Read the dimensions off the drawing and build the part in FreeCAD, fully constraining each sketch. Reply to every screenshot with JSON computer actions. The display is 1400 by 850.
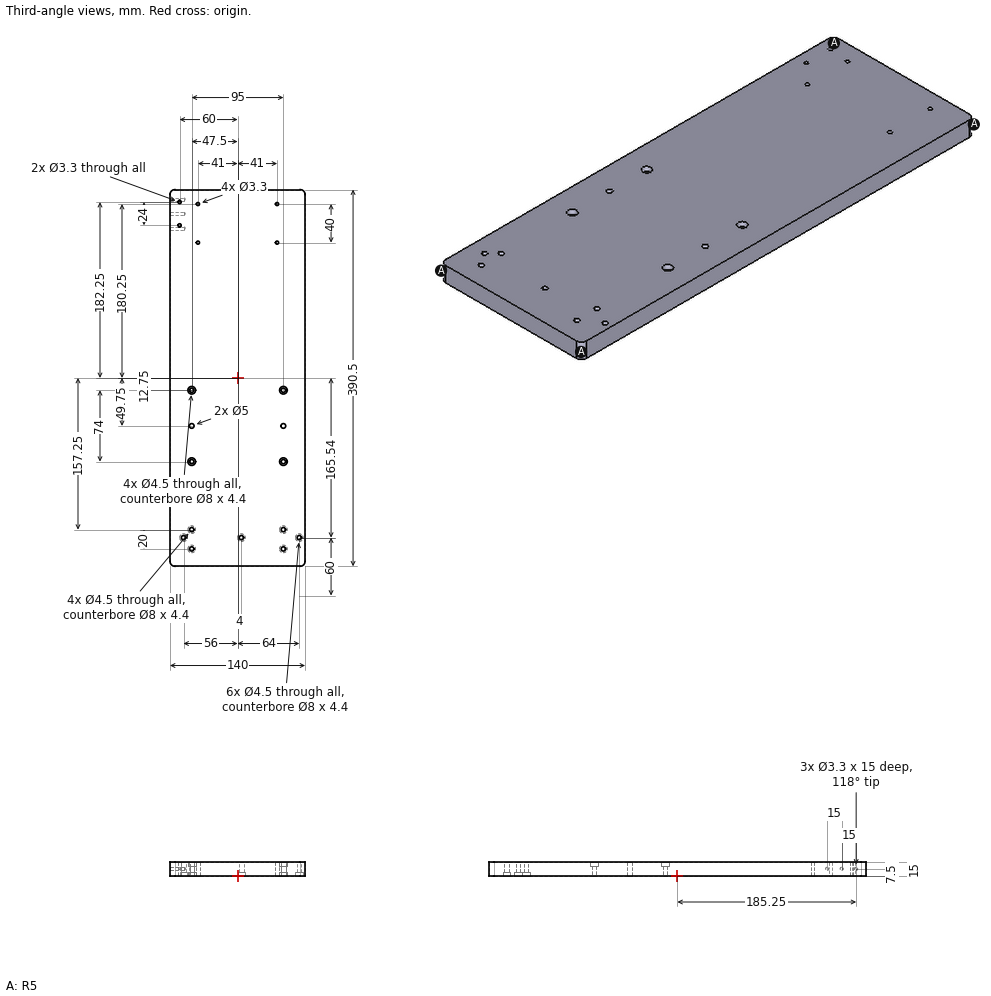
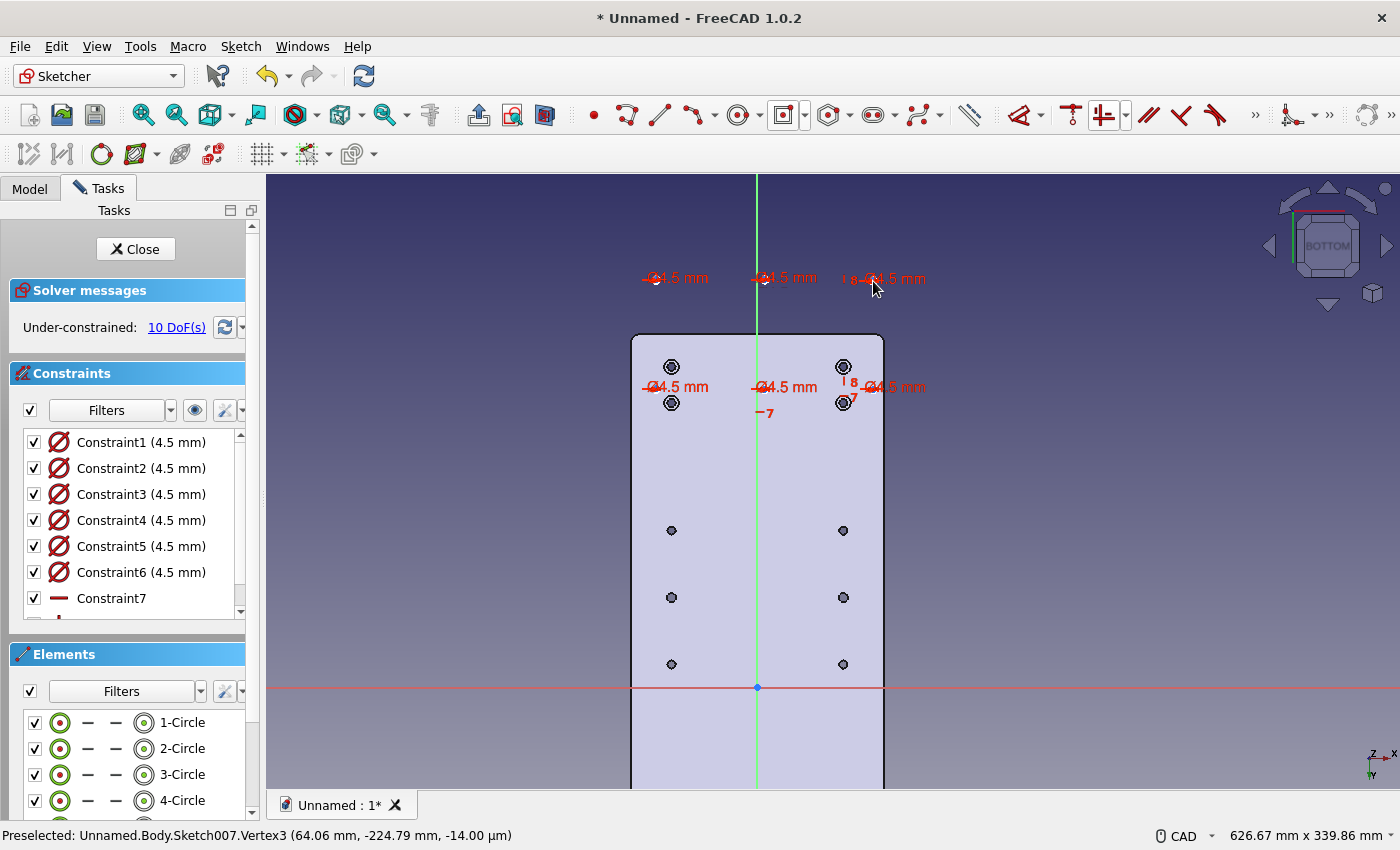
{"action": "left_click", "coordinate": [765, 389]}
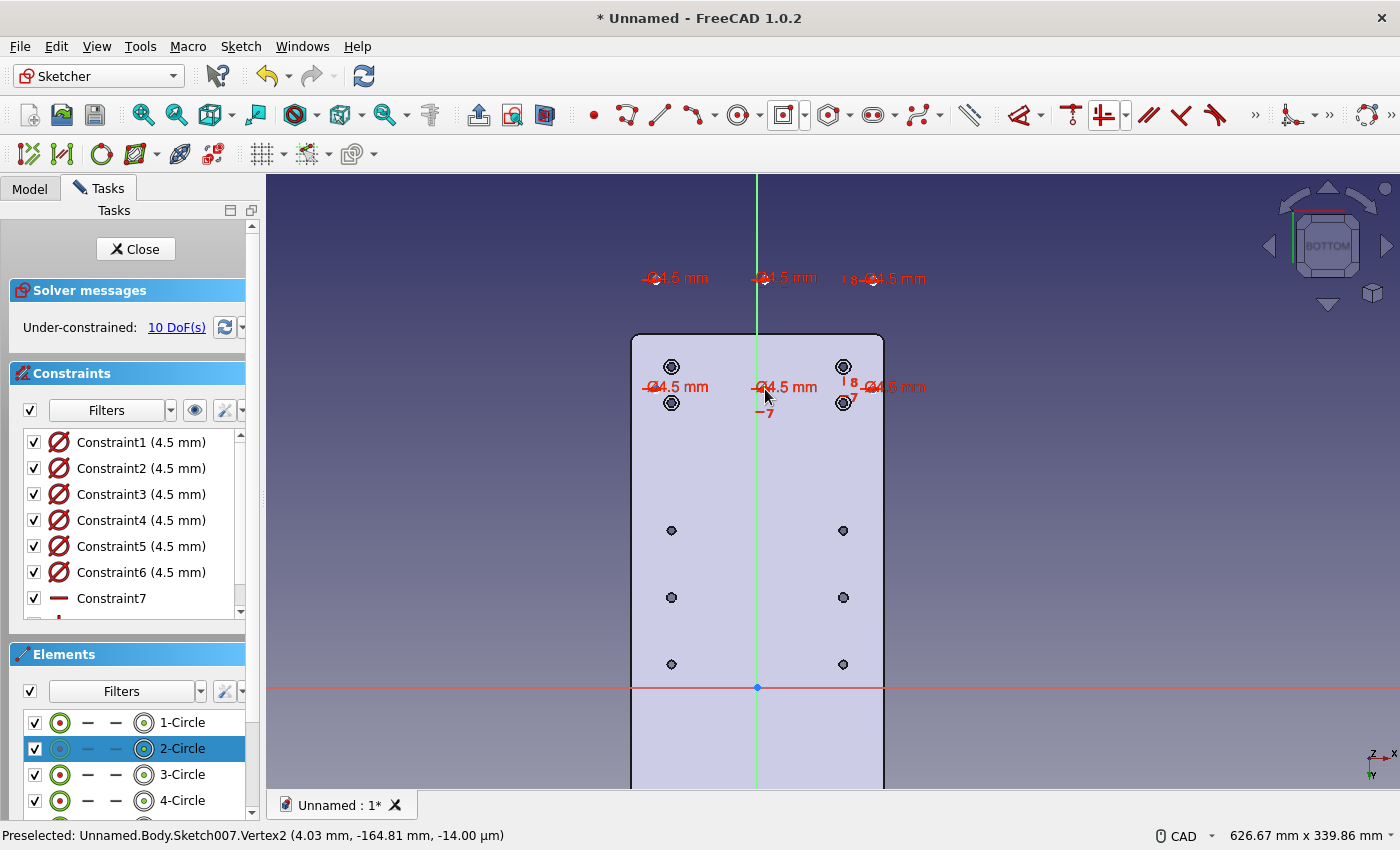
{"action": "left_click", "coordinate": [765, 280]}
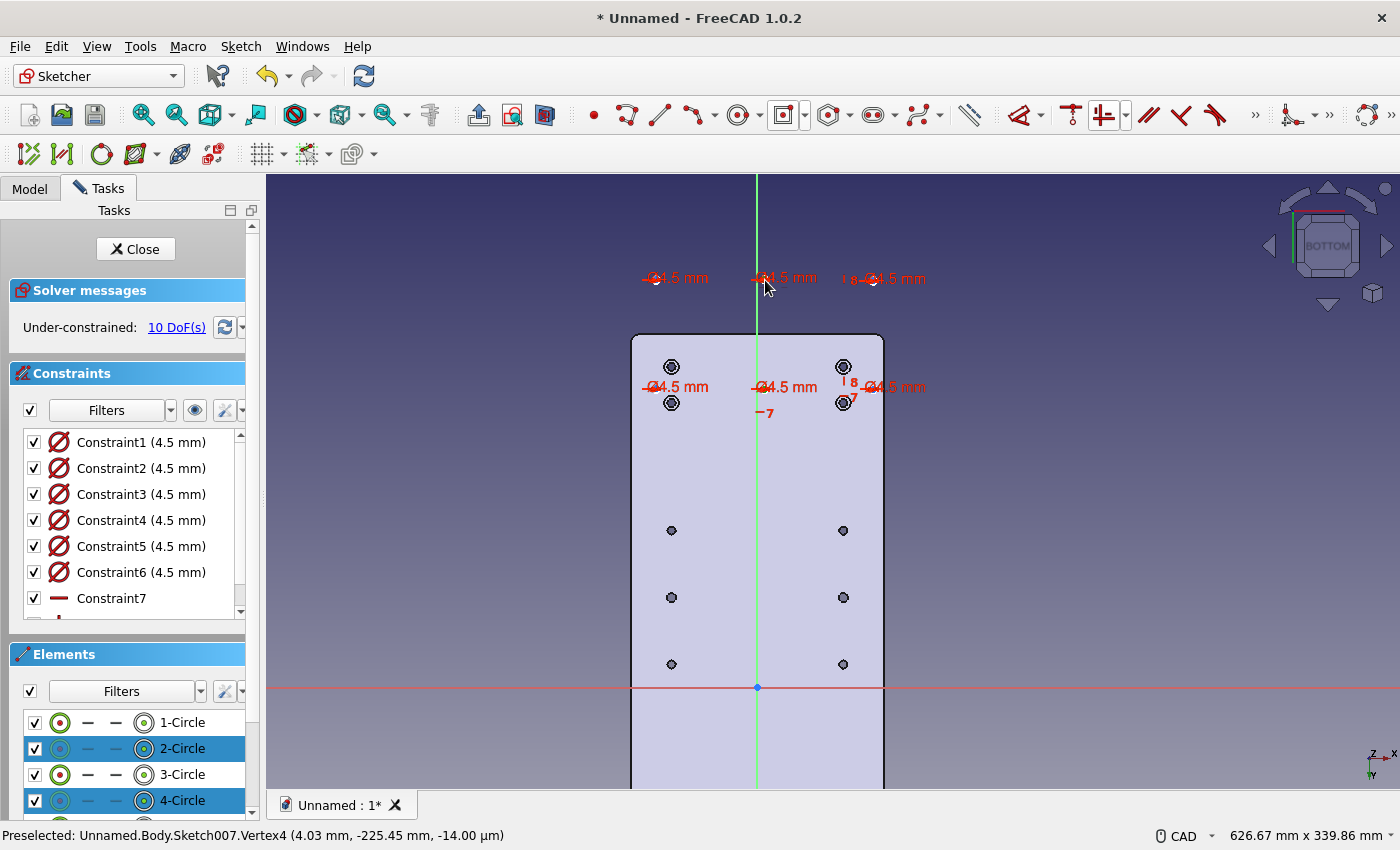
{"action": "key", "text": "v"}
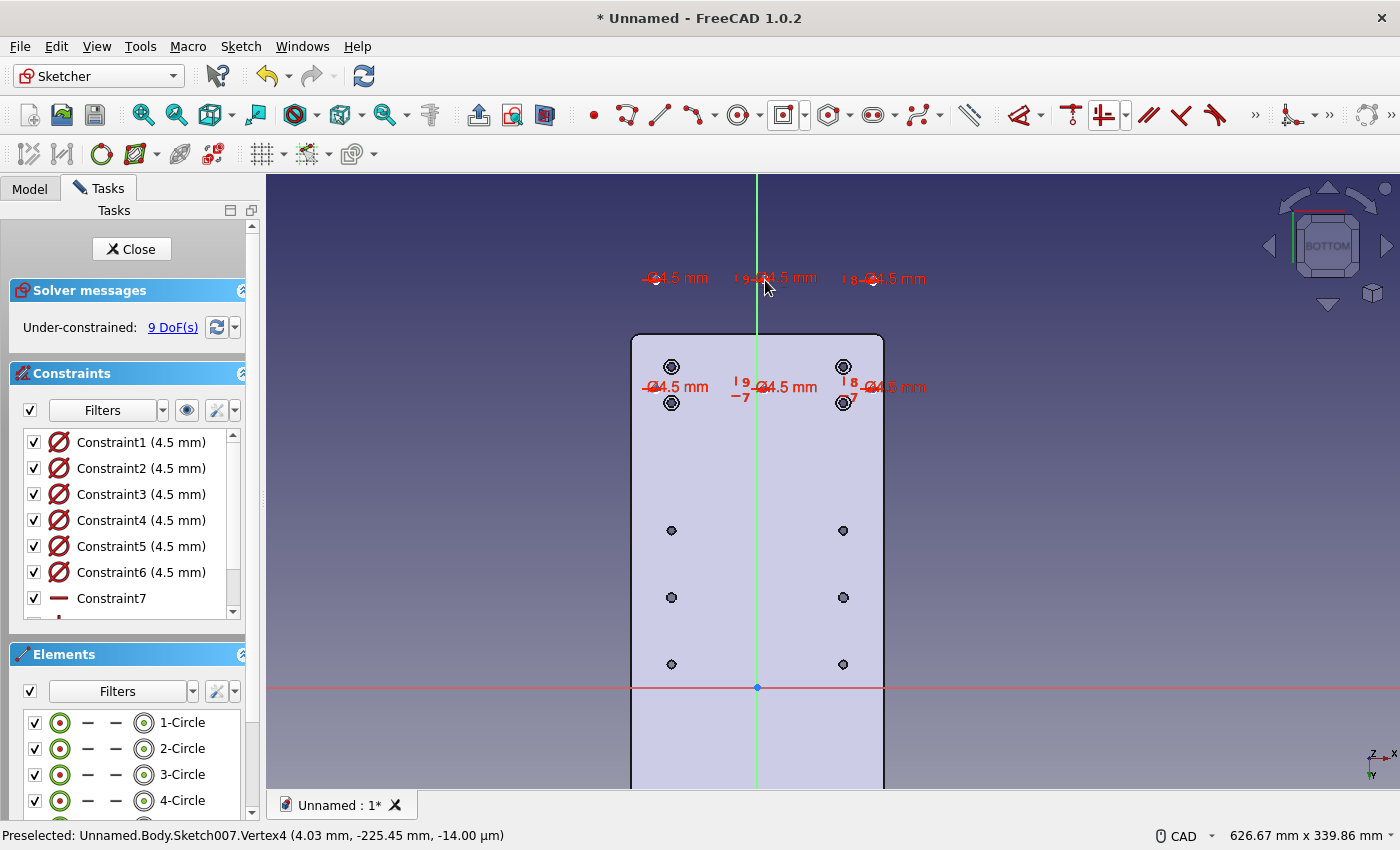
{"action": "left_click", "coordinate": [873, 281]}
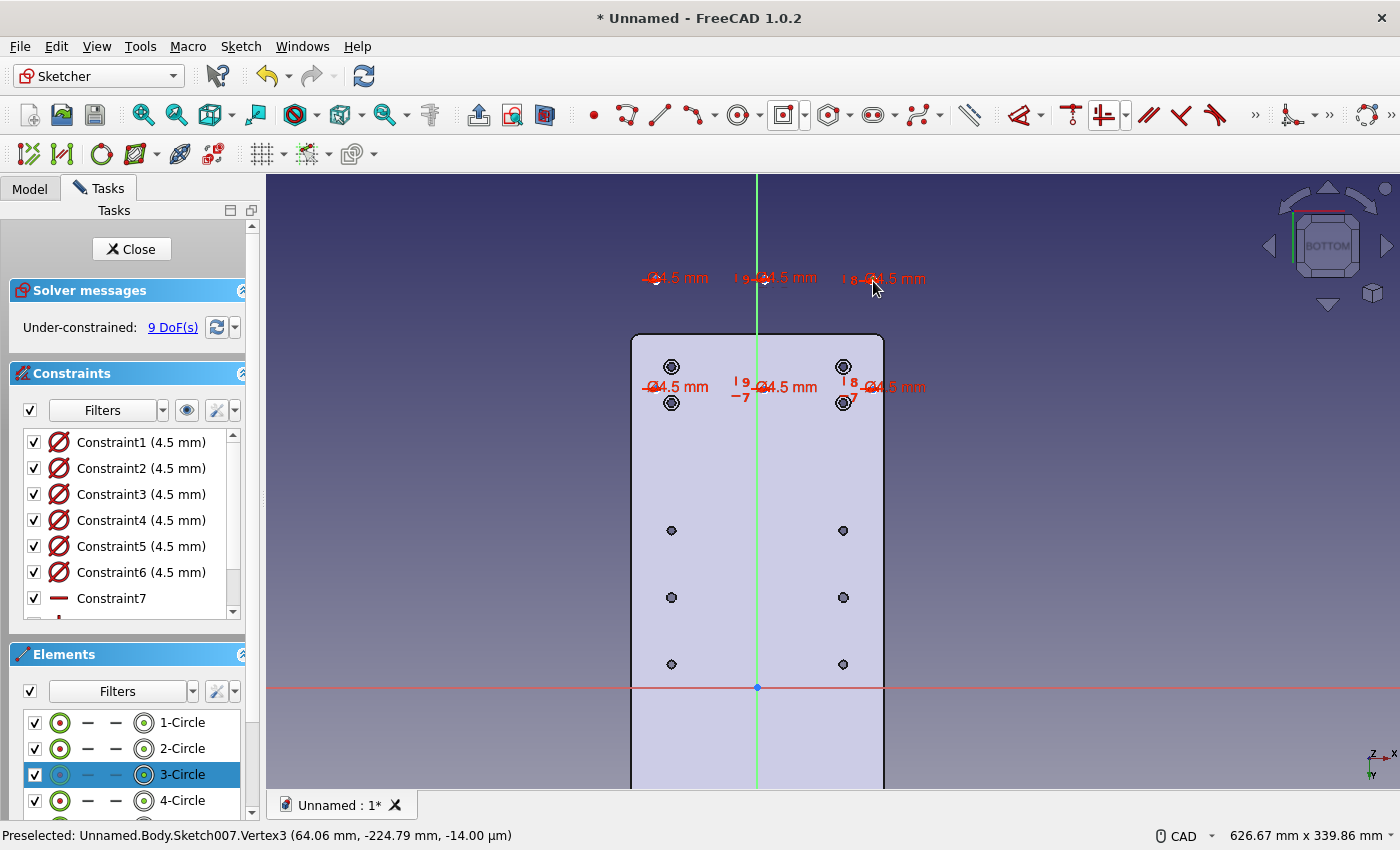
{"action": "left_click", "coordinate": [765, 280]}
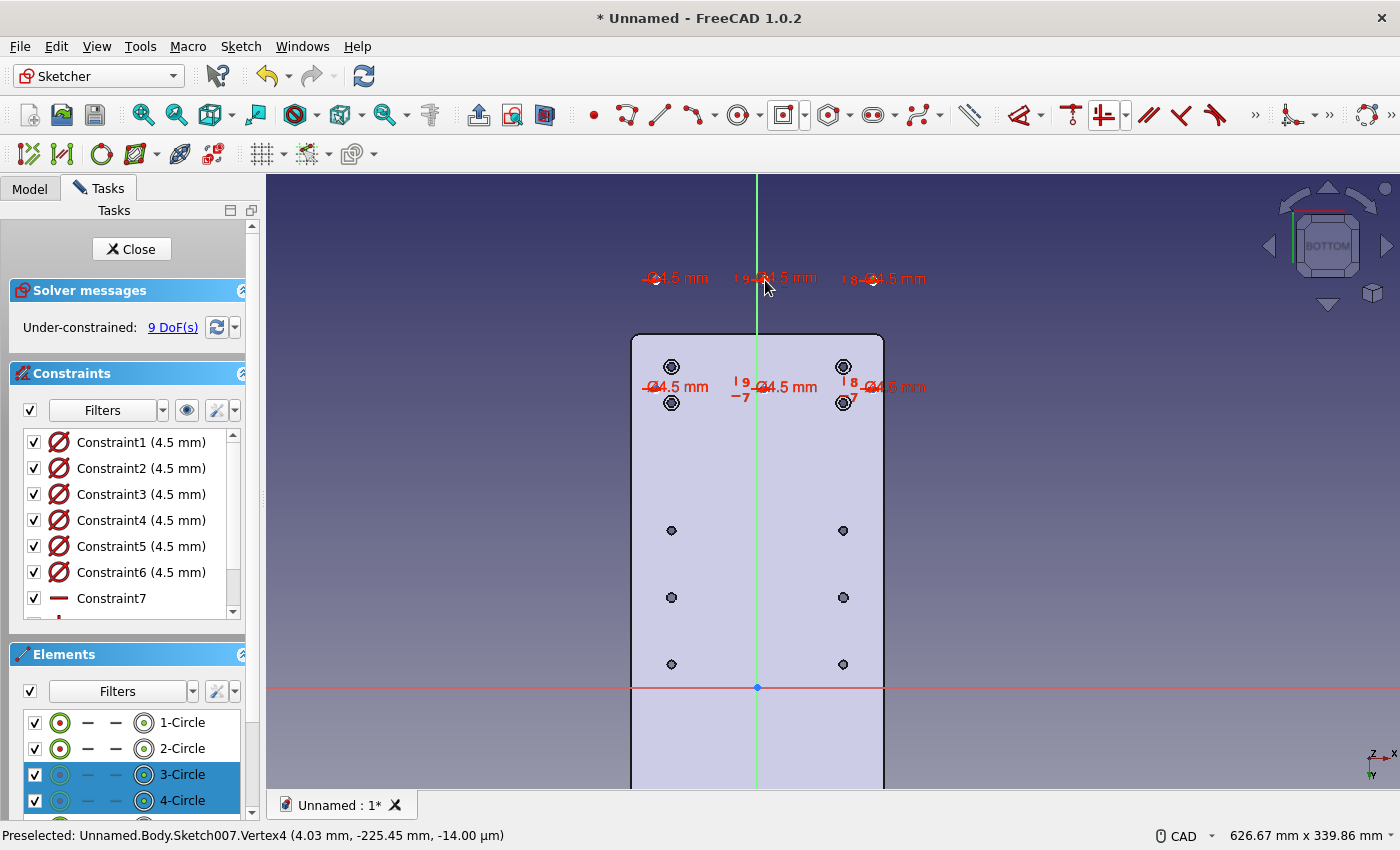
{"action": "left_click", "coordinate": [1126, 116]}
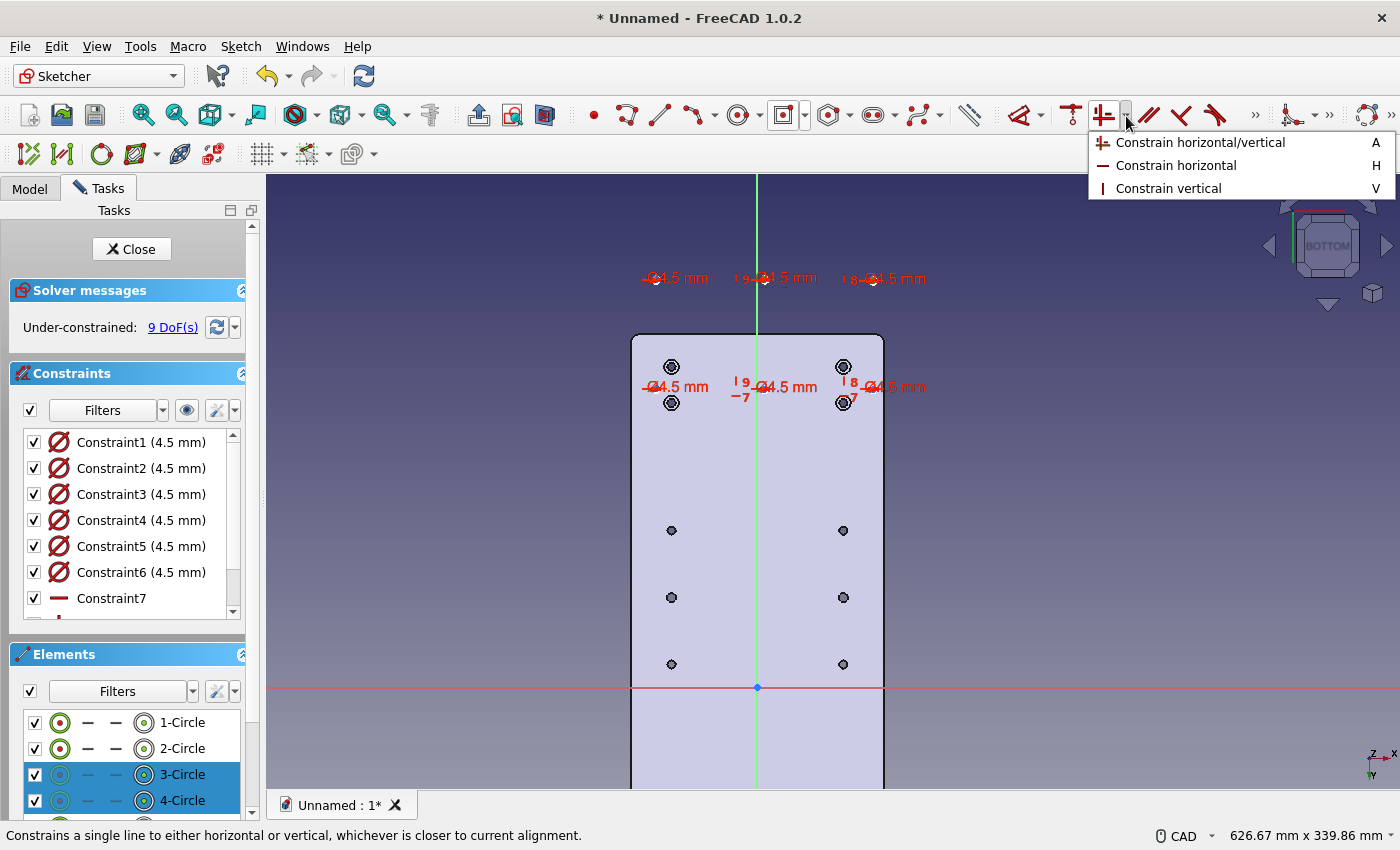
{"action": "left_click", "coordinate": [1242, 166]}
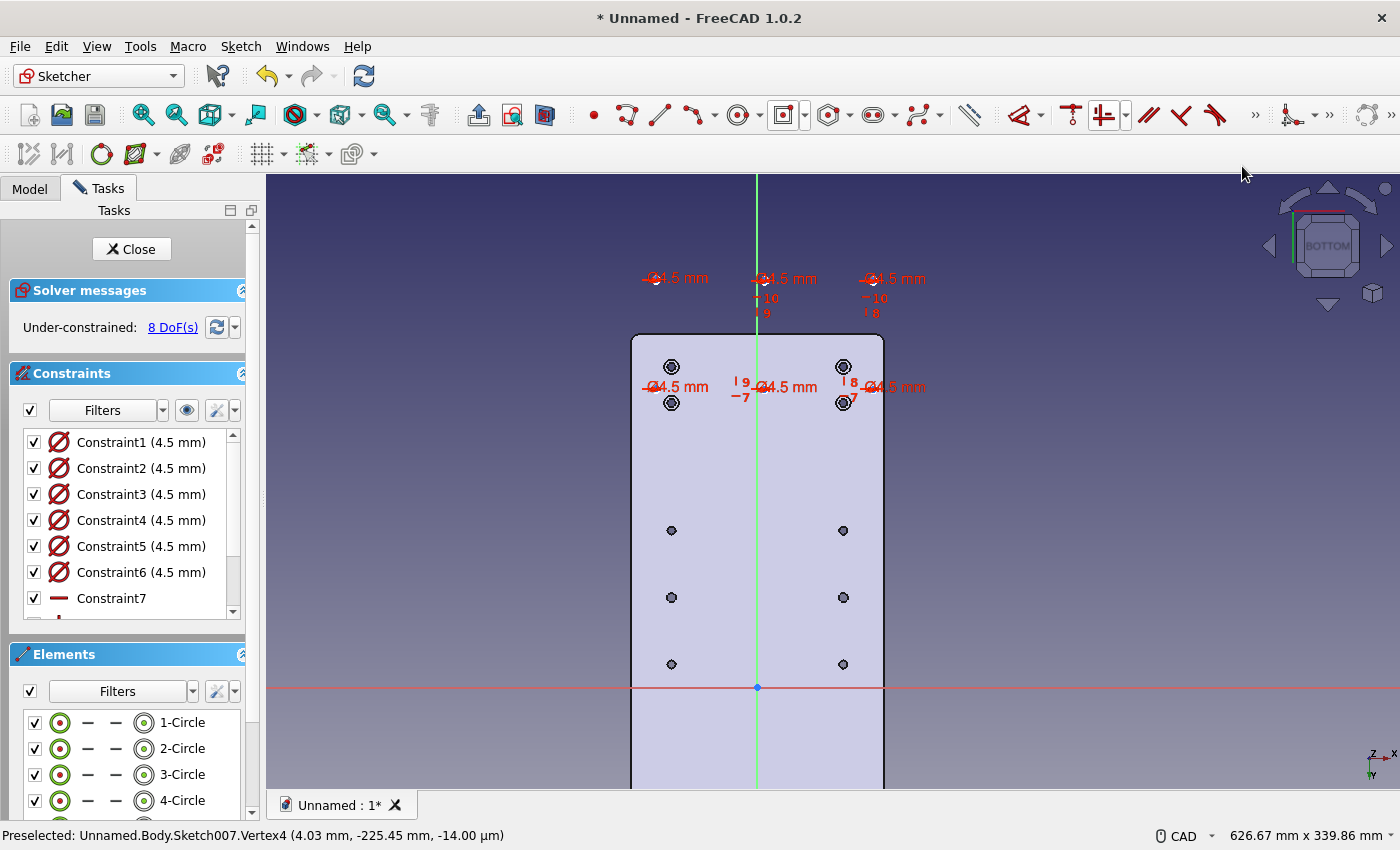
{"action": "left_click", "coordinate": [765, 389]}